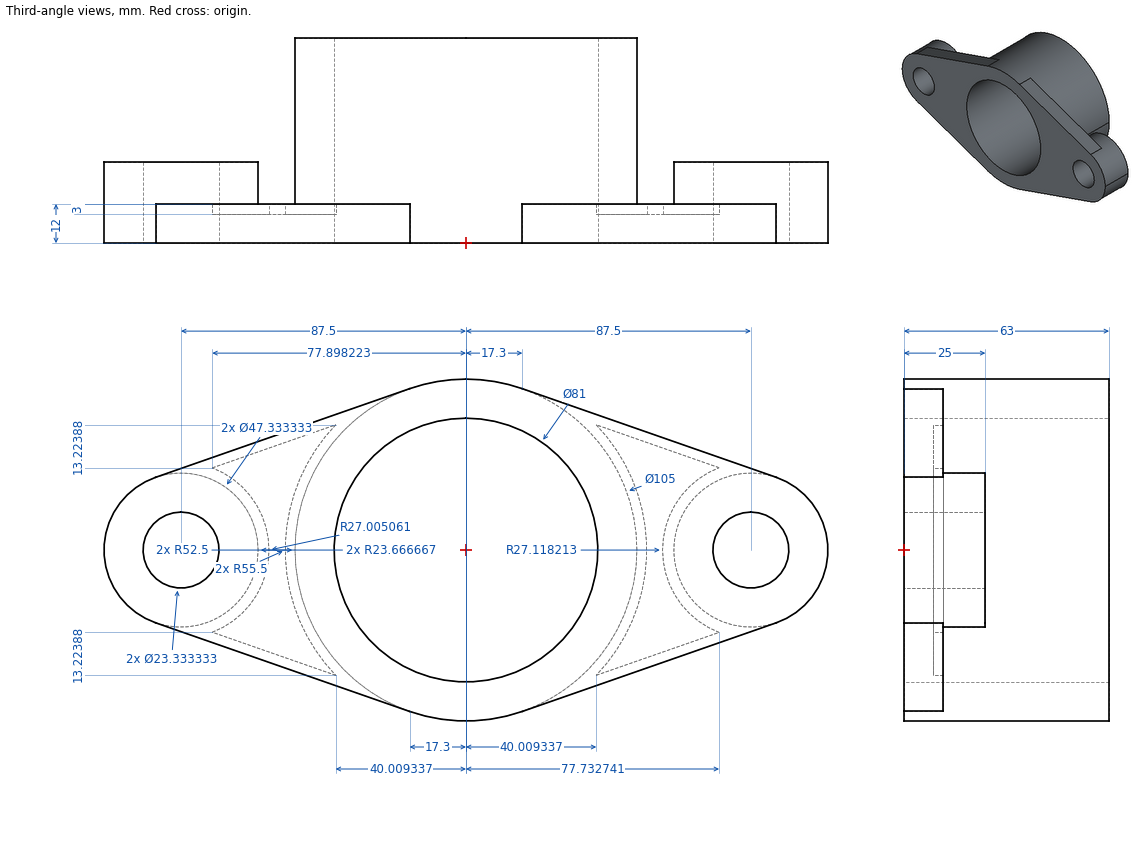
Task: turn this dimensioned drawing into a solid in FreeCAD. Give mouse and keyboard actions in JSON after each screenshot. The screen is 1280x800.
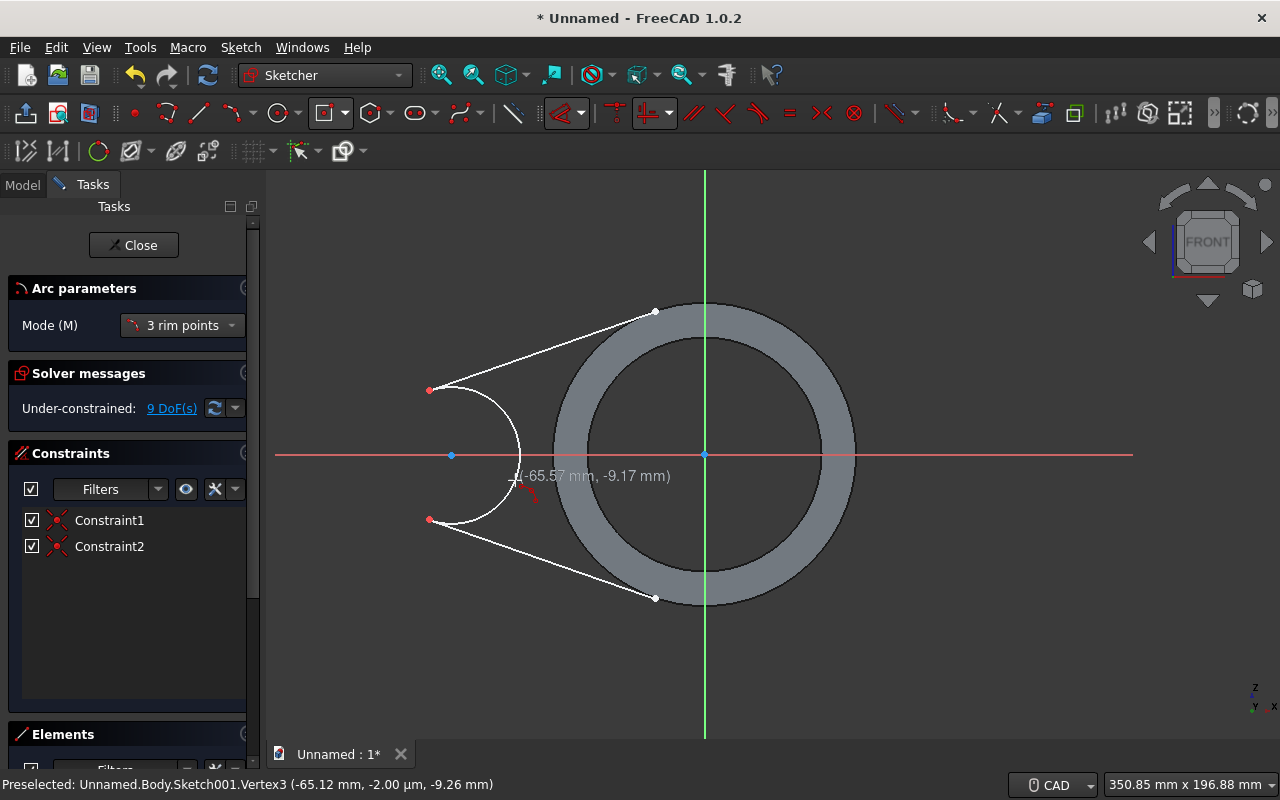
{"action": "left_click", "coordinate": [655, 312]}
{"action": "left_click", "coordinate": [655, 599]}
{"action": "left_click", "coordinate": [557, 417]}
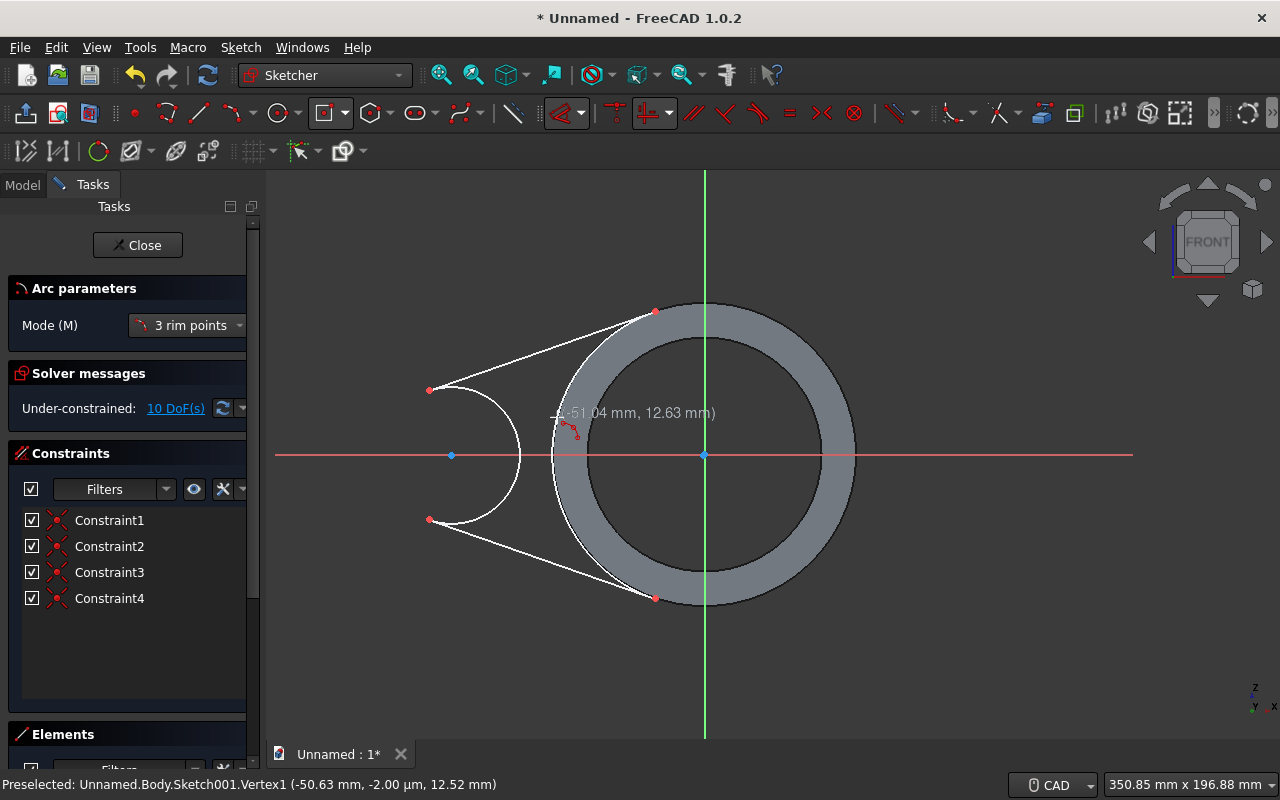
{"action": "key", "text": "g l"}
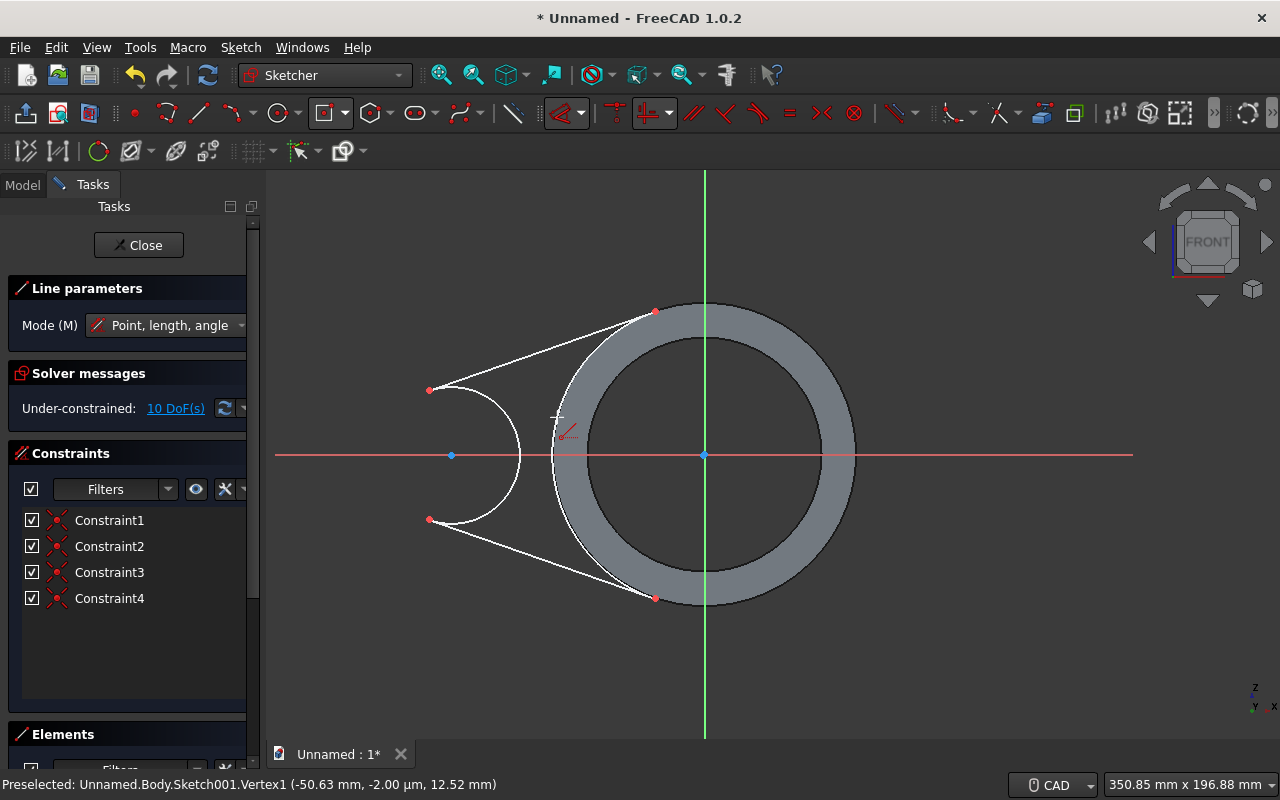
{"action": "left_click", "coordinate": [980, 519]}
{"action": "left_click", "coordinate": [755, 598]}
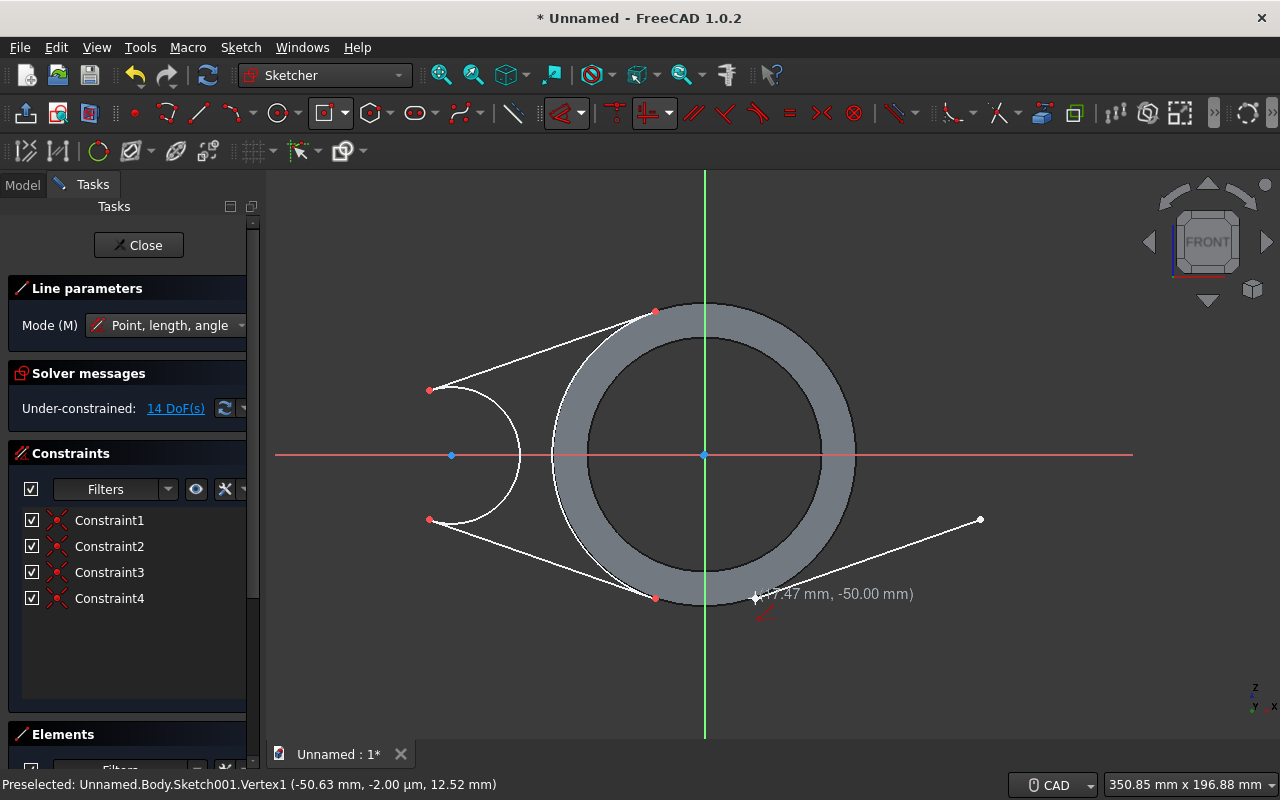
{"action": "left_click", "coordinate": [755, 311]}
{"action": "left_click", "coordinate": [980, 390]}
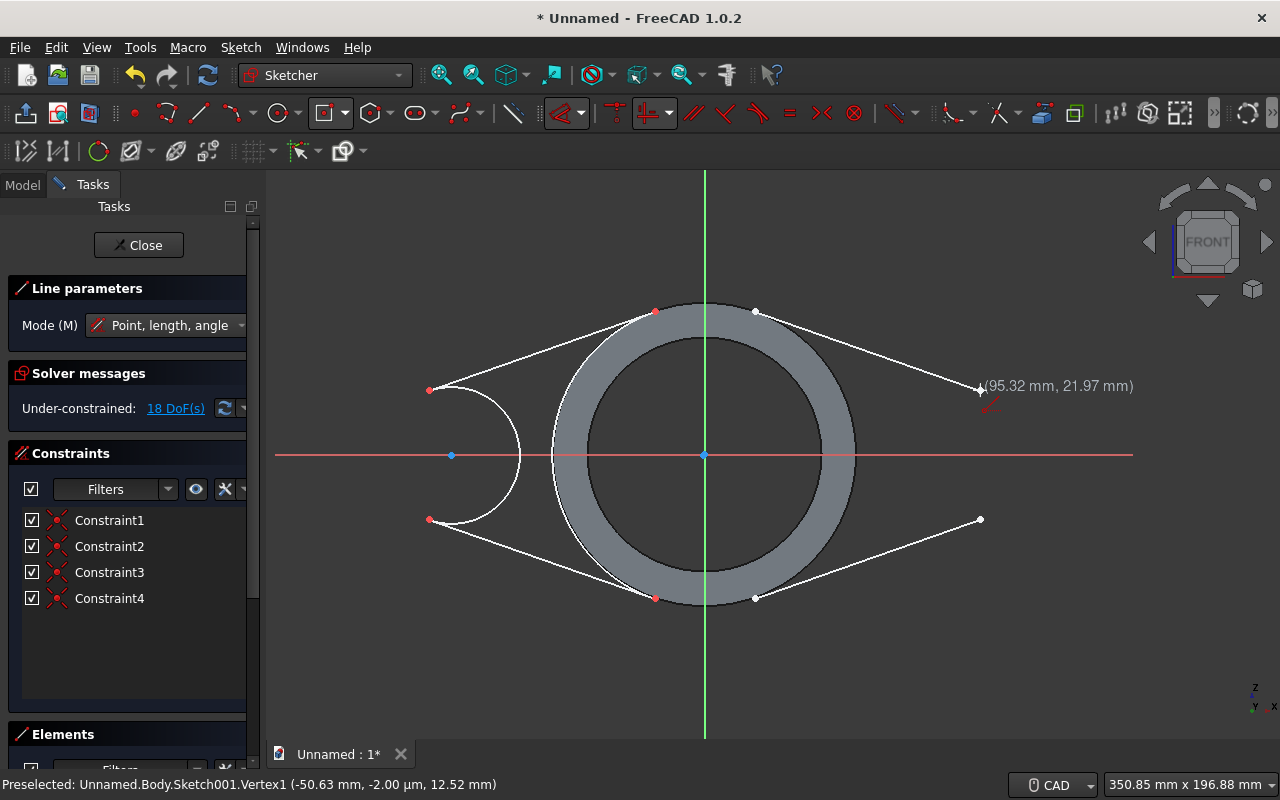
{"action": "key", "text": "g 3 a"}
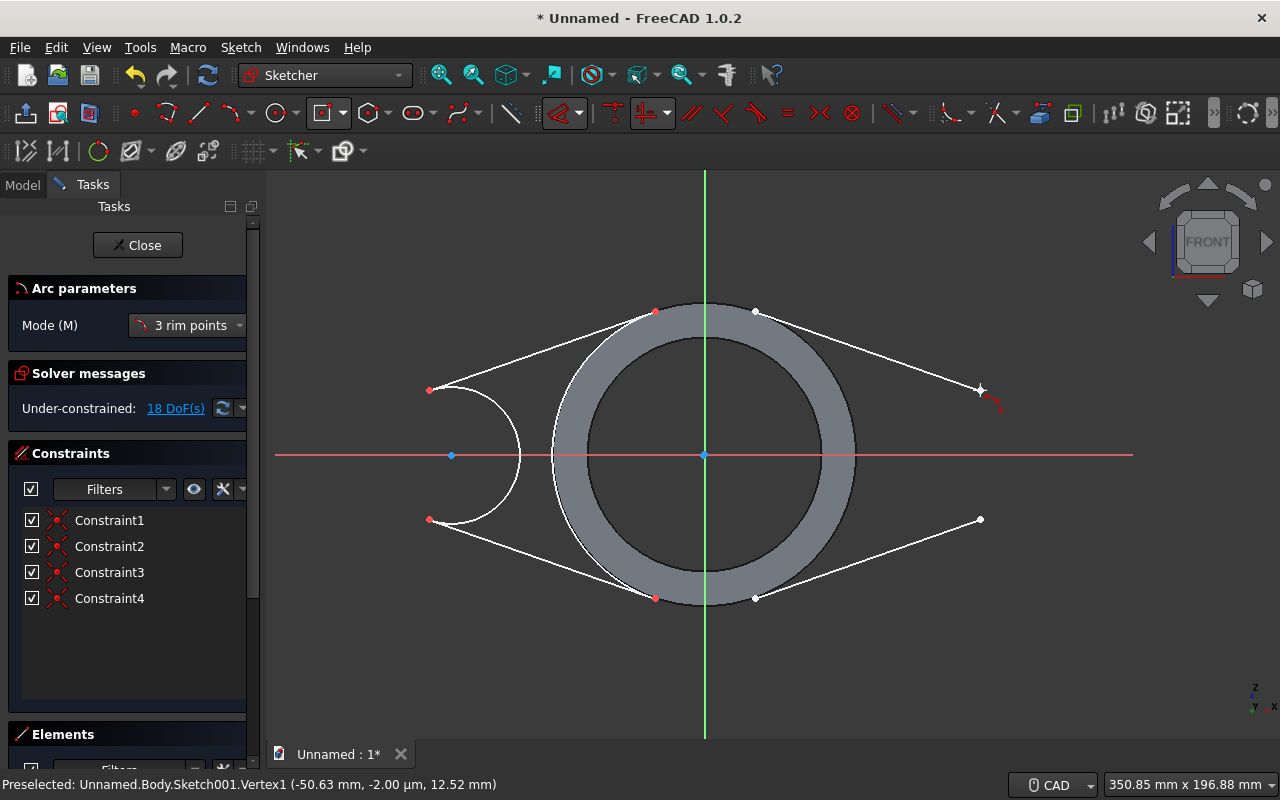
{"action": "left_click", "coordinate": [755, 599]}
{"action": "left_click", "coordinate": [755, 312]}
{"action": "left_click", "coordinate": [852, 492]}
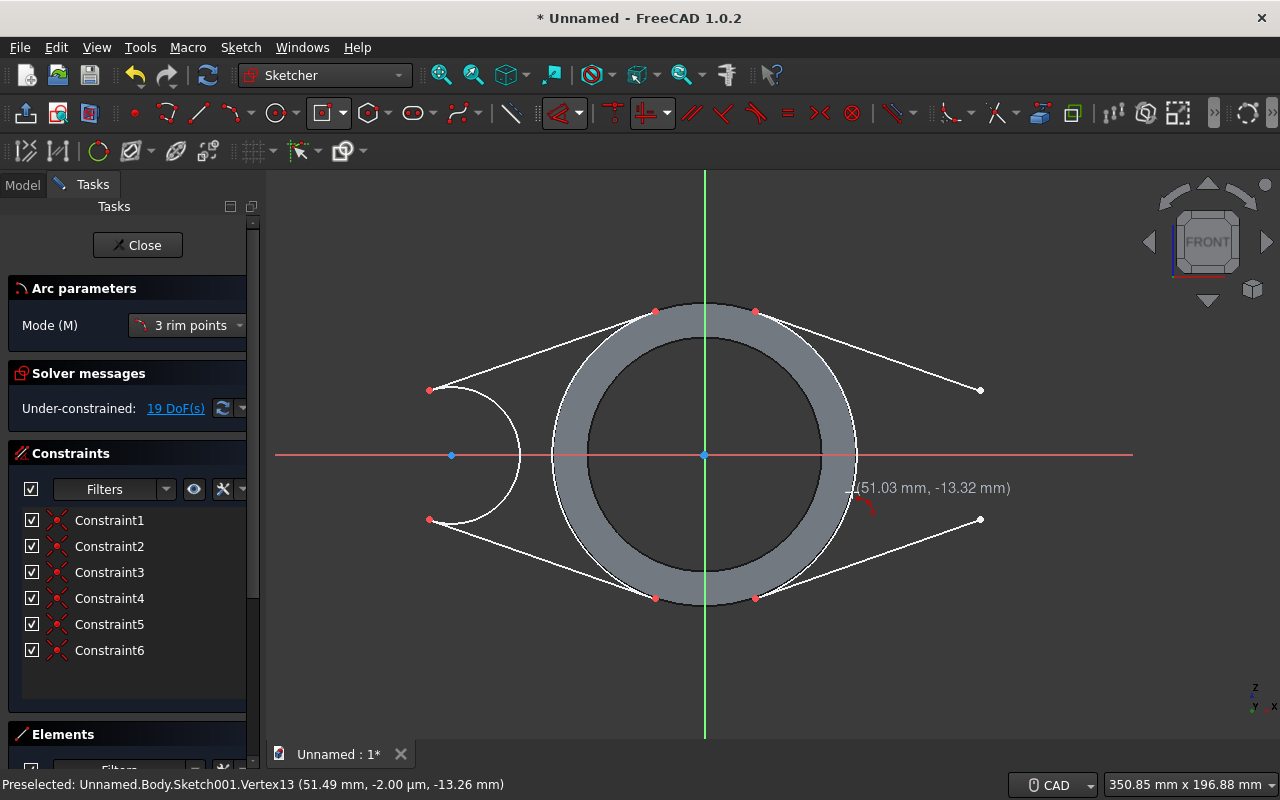
{"action": "left_click", "coordinate": [980, 391]}
{"action": "left_click", "coordinate": [980, 520]}
{"action": "left_click", "coordinate": [894, 429]}
{"action": "key", "text": "Escape"}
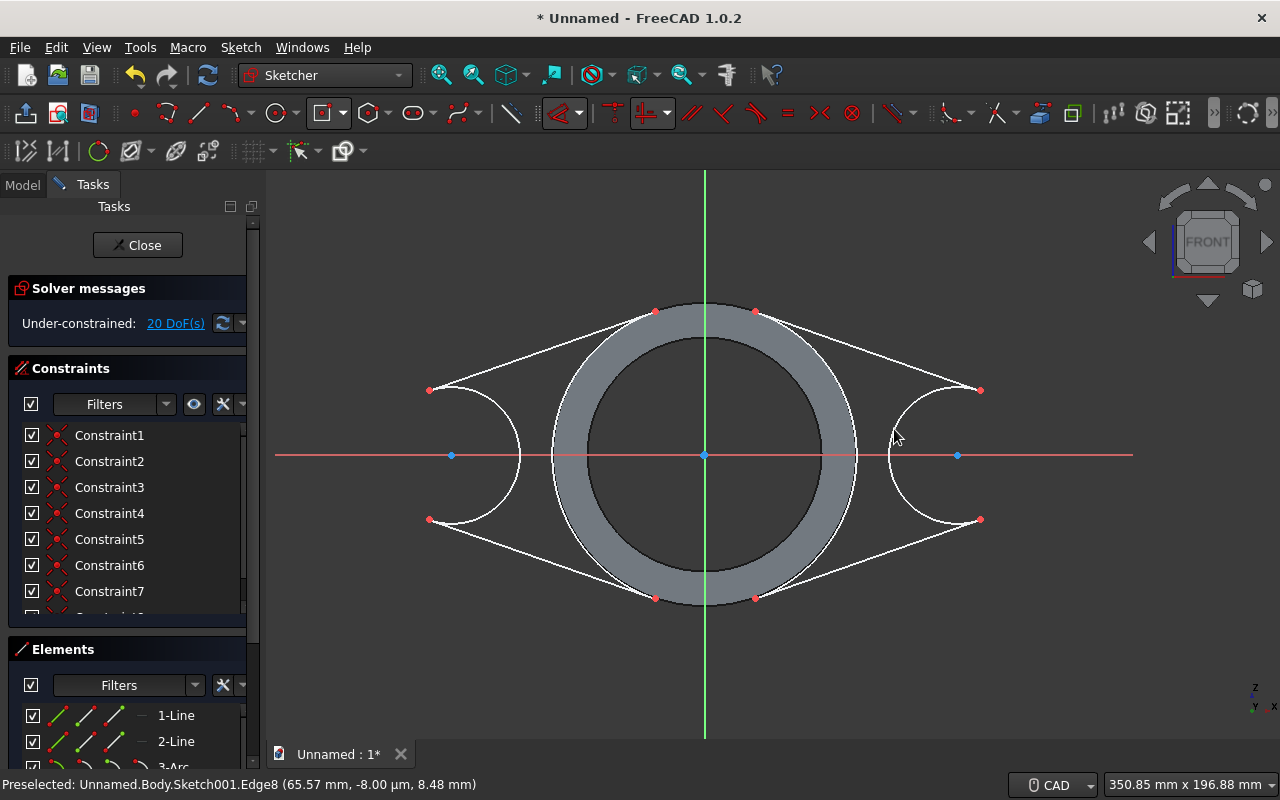
{"action": "left_click", "coordinate": [587, 575]}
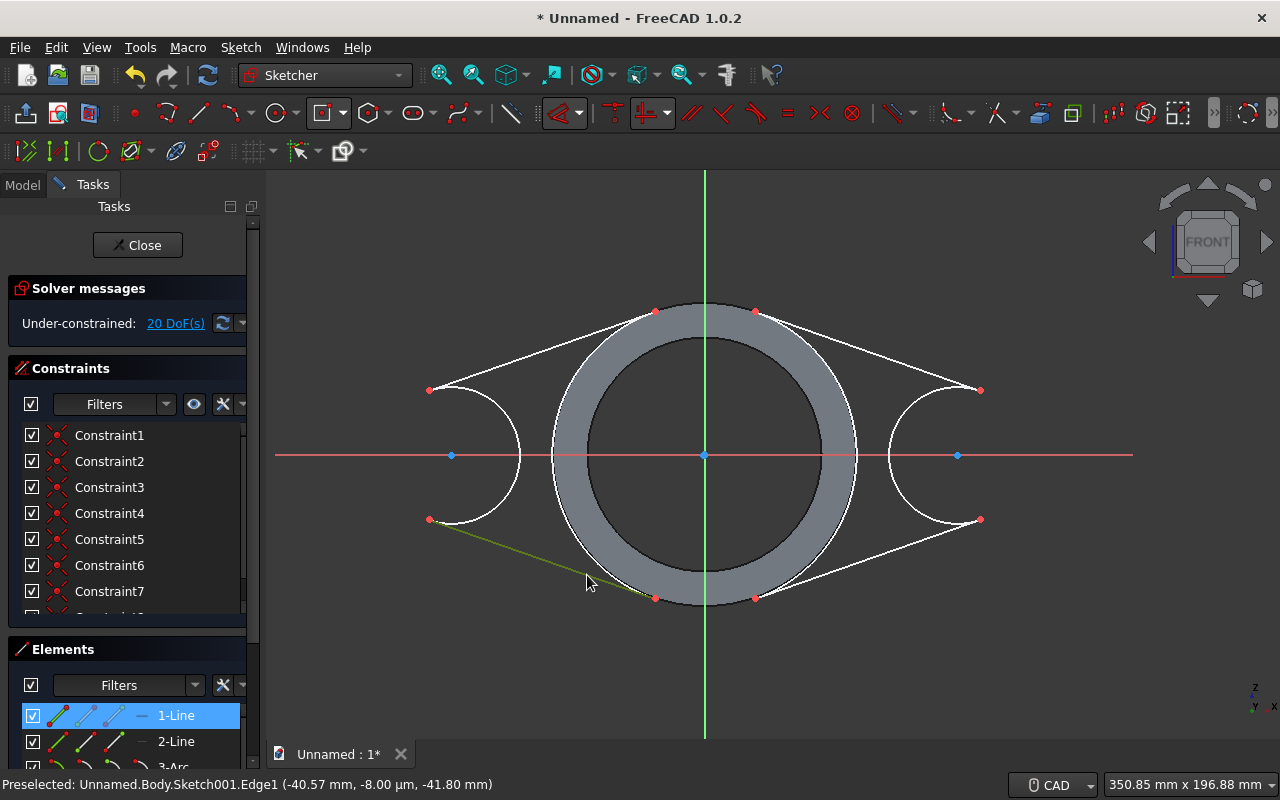
{"action": "left_click", "coordinate": [501, 503]}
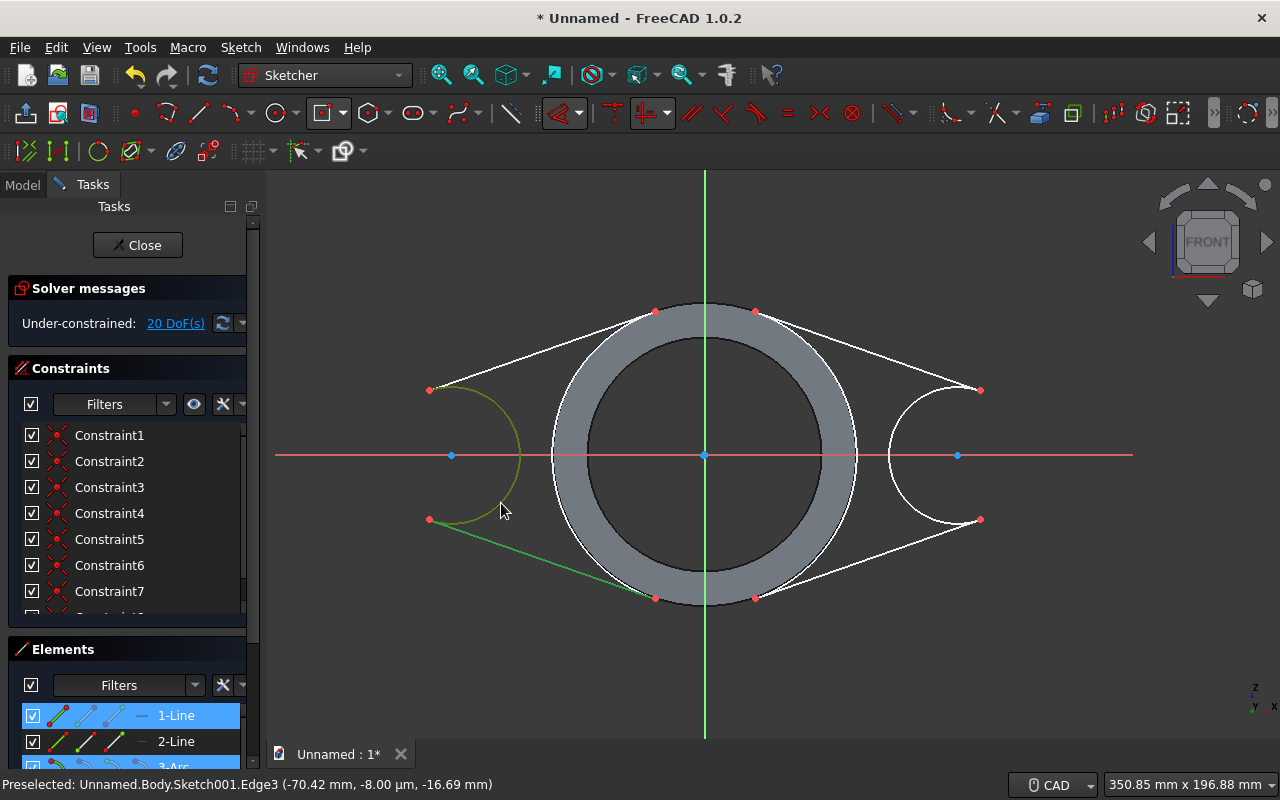
{"action": "key", "text": "t"}